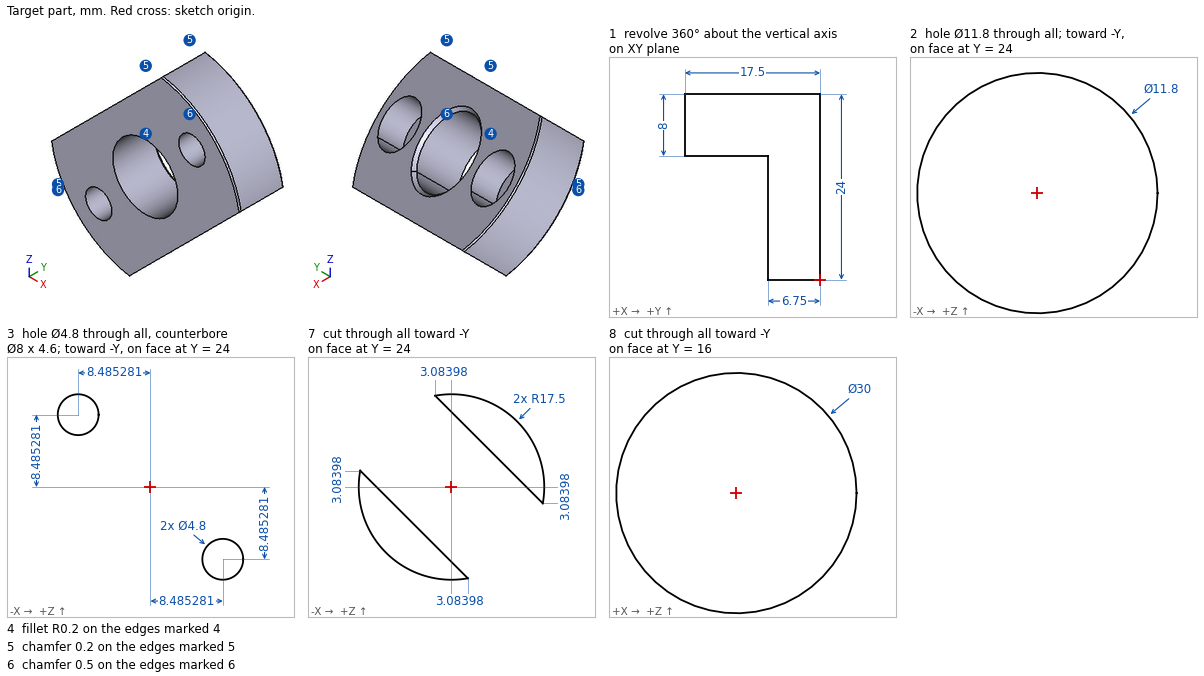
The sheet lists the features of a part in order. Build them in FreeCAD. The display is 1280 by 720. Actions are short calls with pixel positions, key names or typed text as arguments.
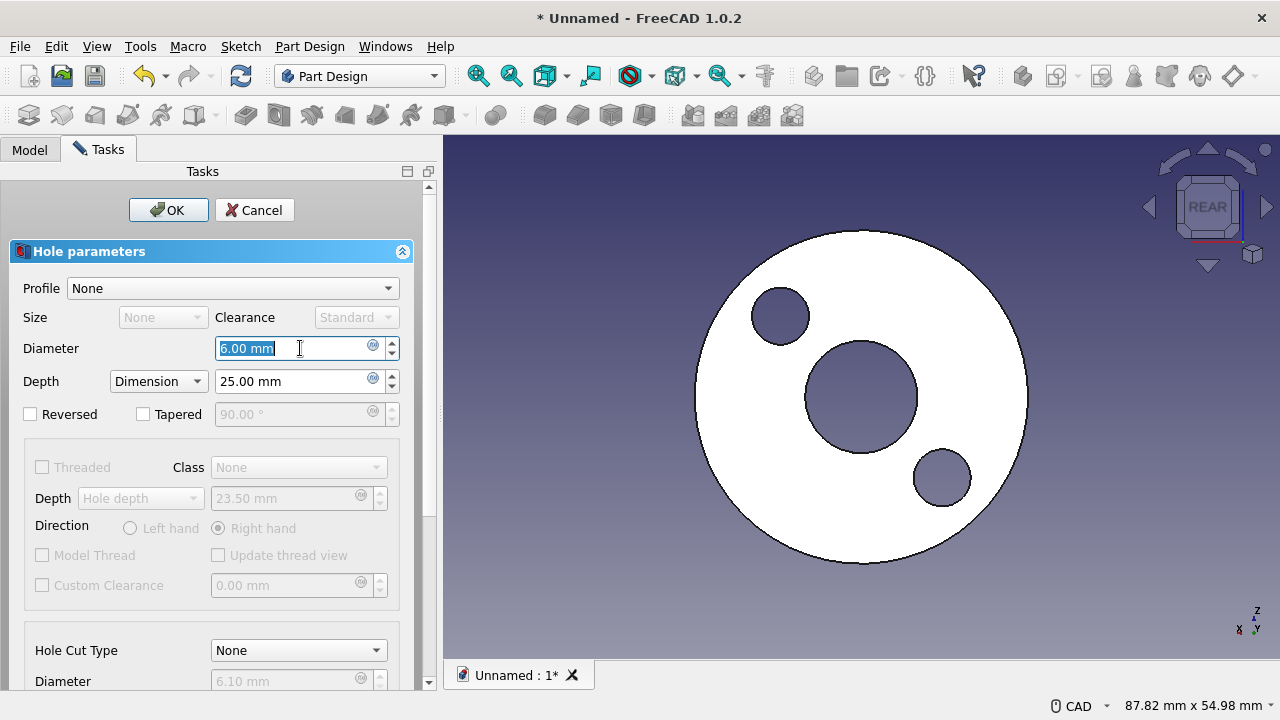
text(4.8)
key(Tab)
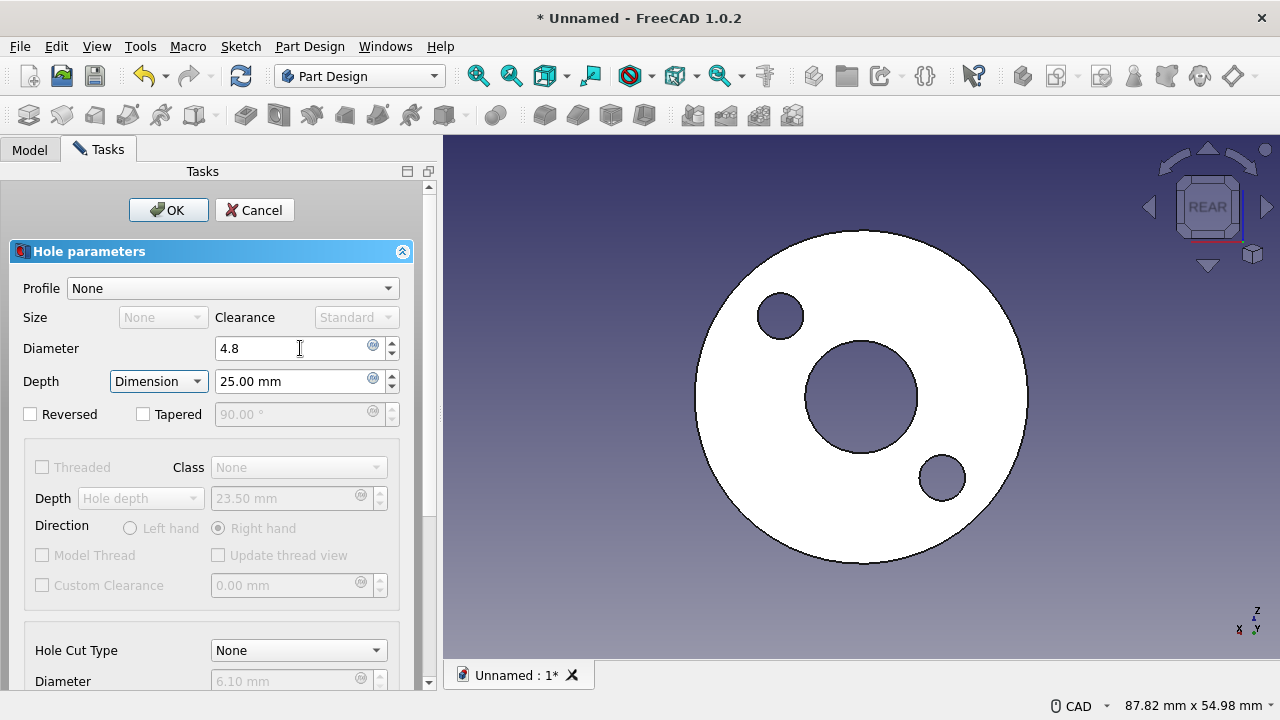
click(160, 382)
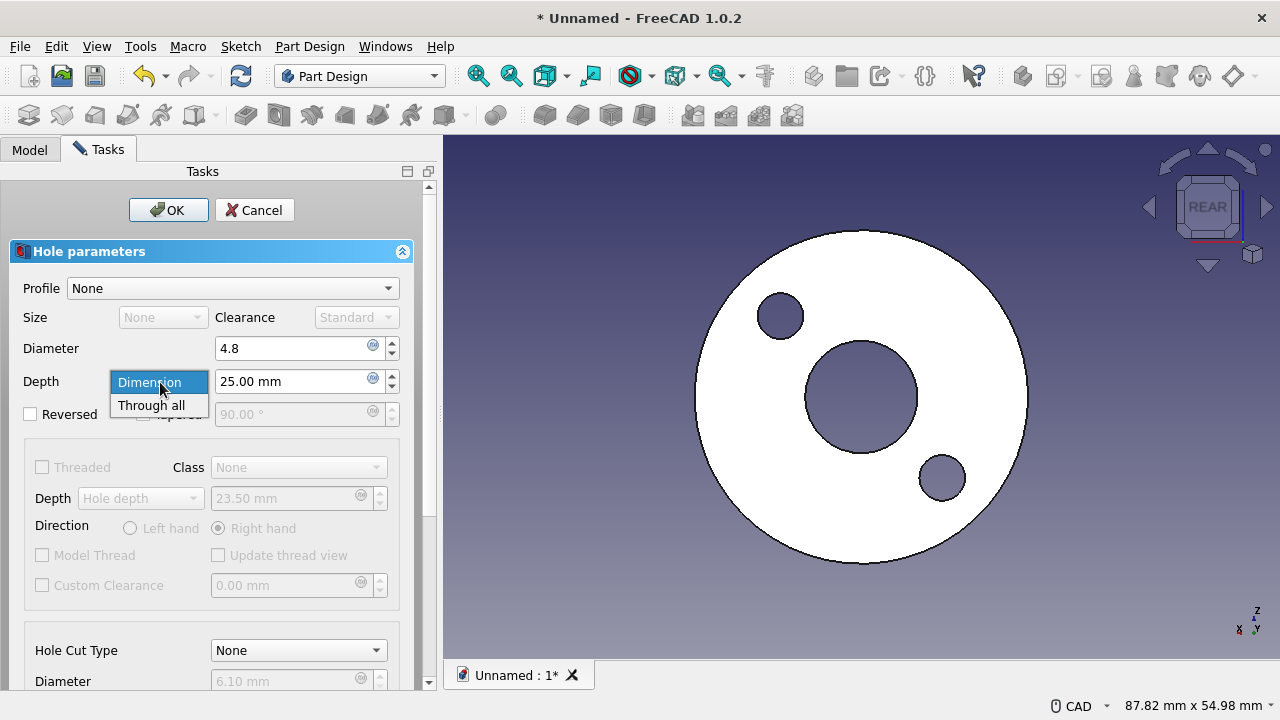
click(158, 406)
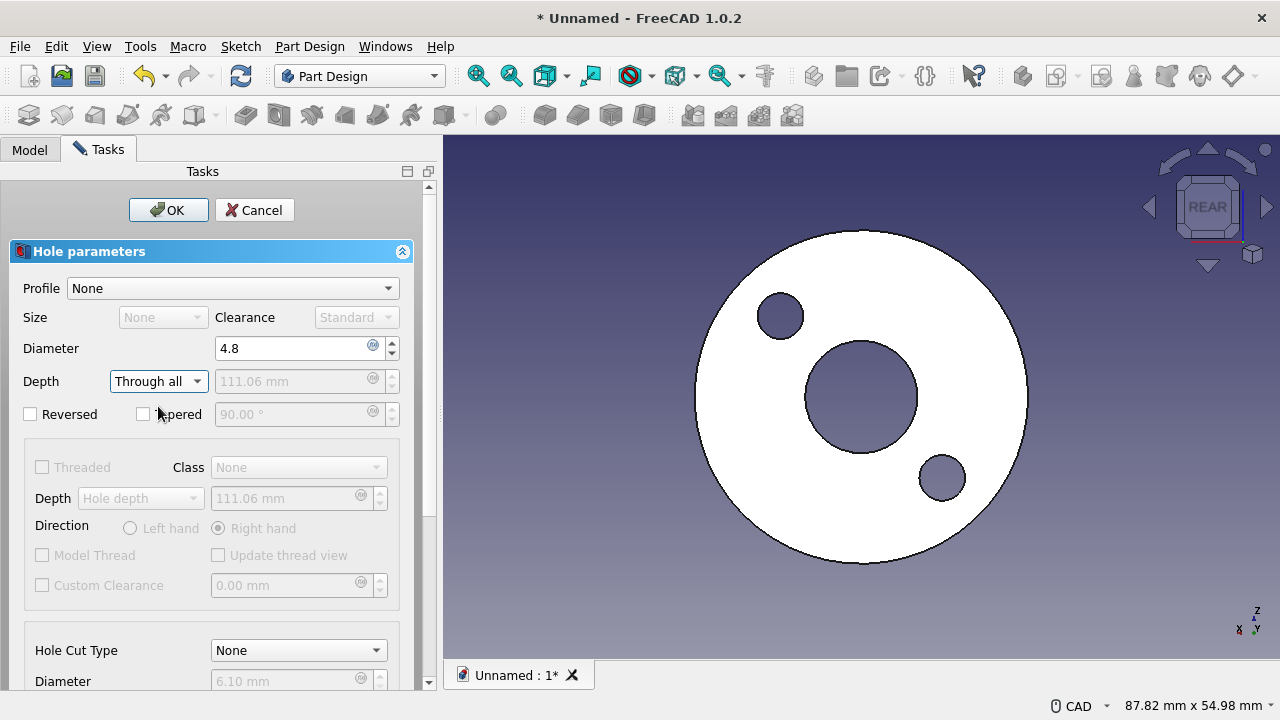
click(300, 650)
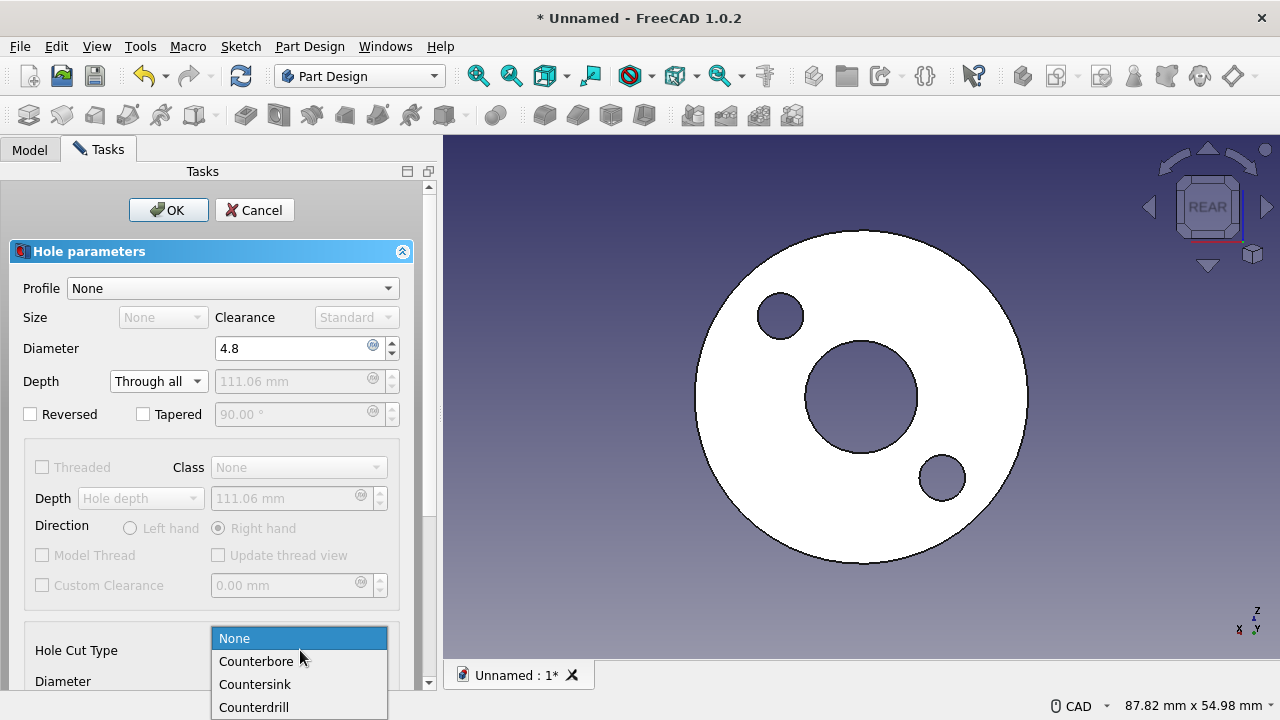
click(298, 662)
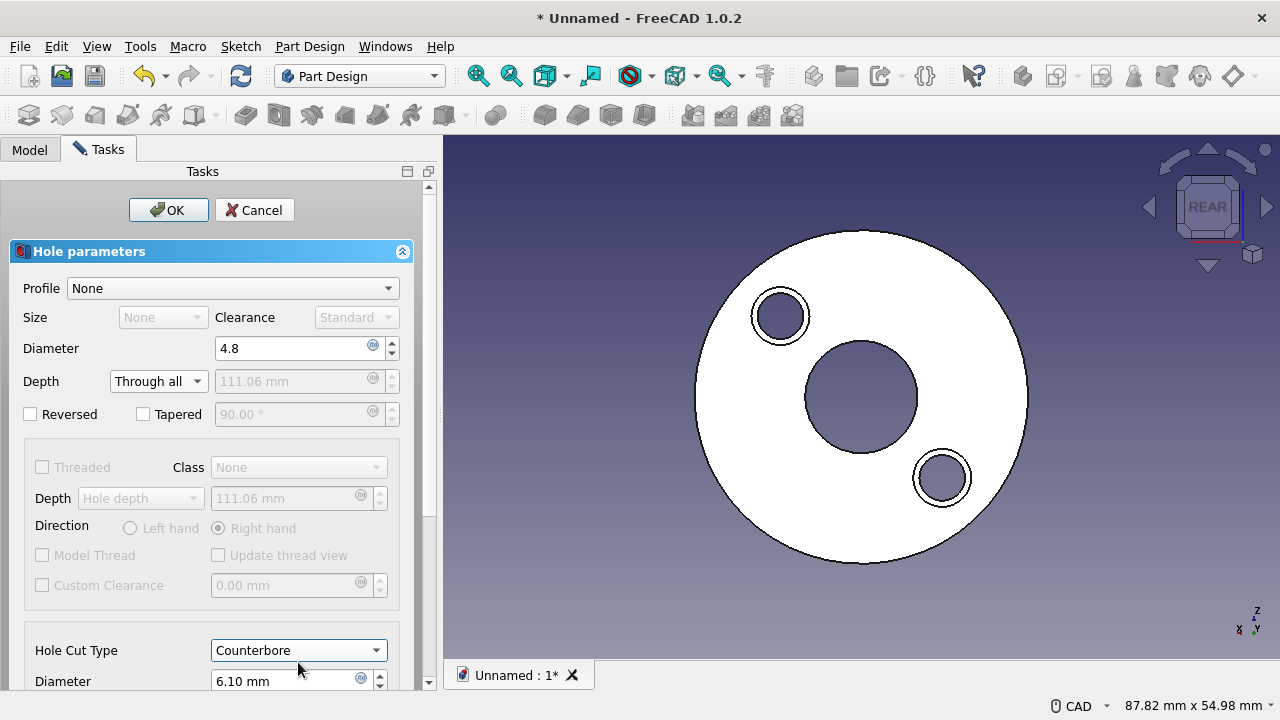
scroll(429, 436, down, 2)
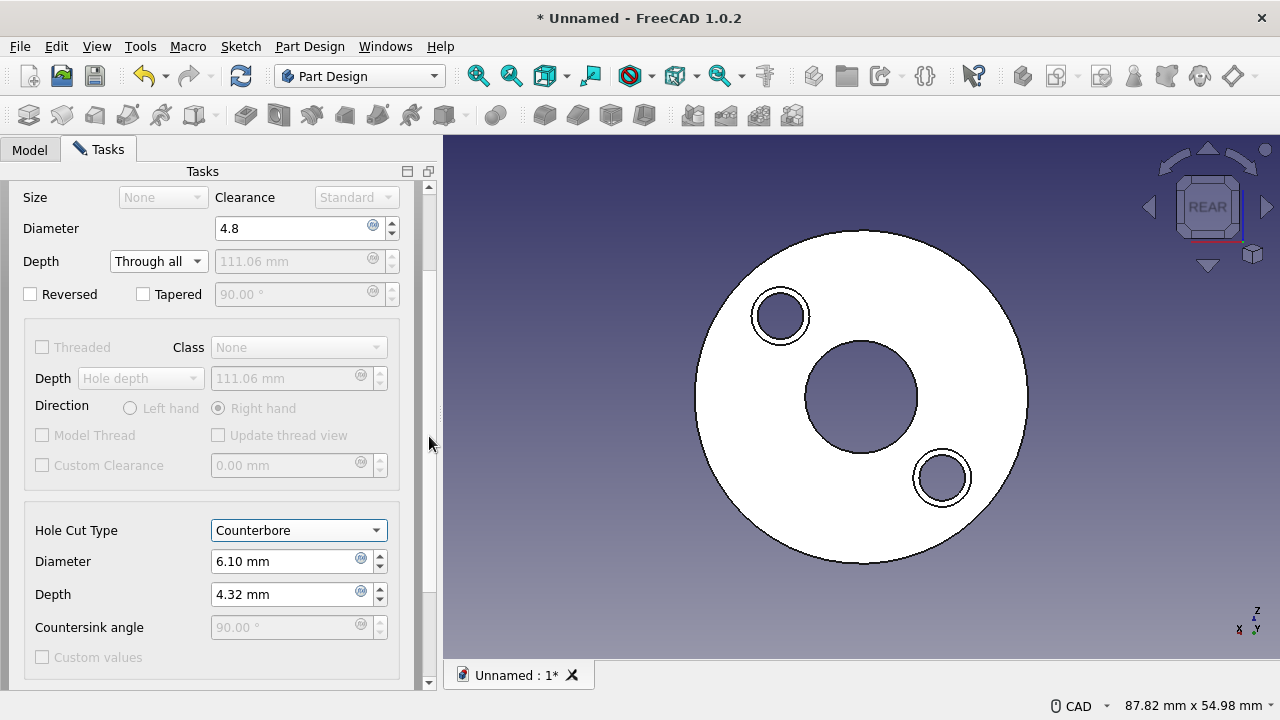
triple_click(292, 562)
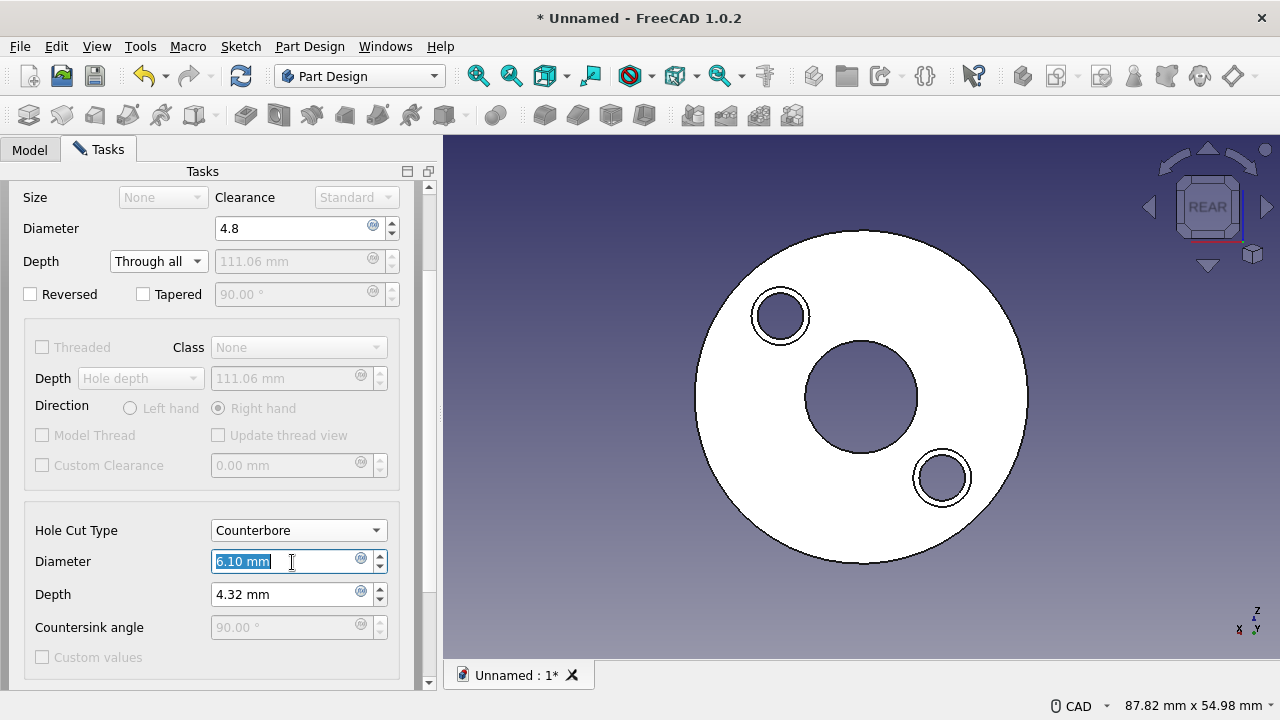
text(8)
key(Tab)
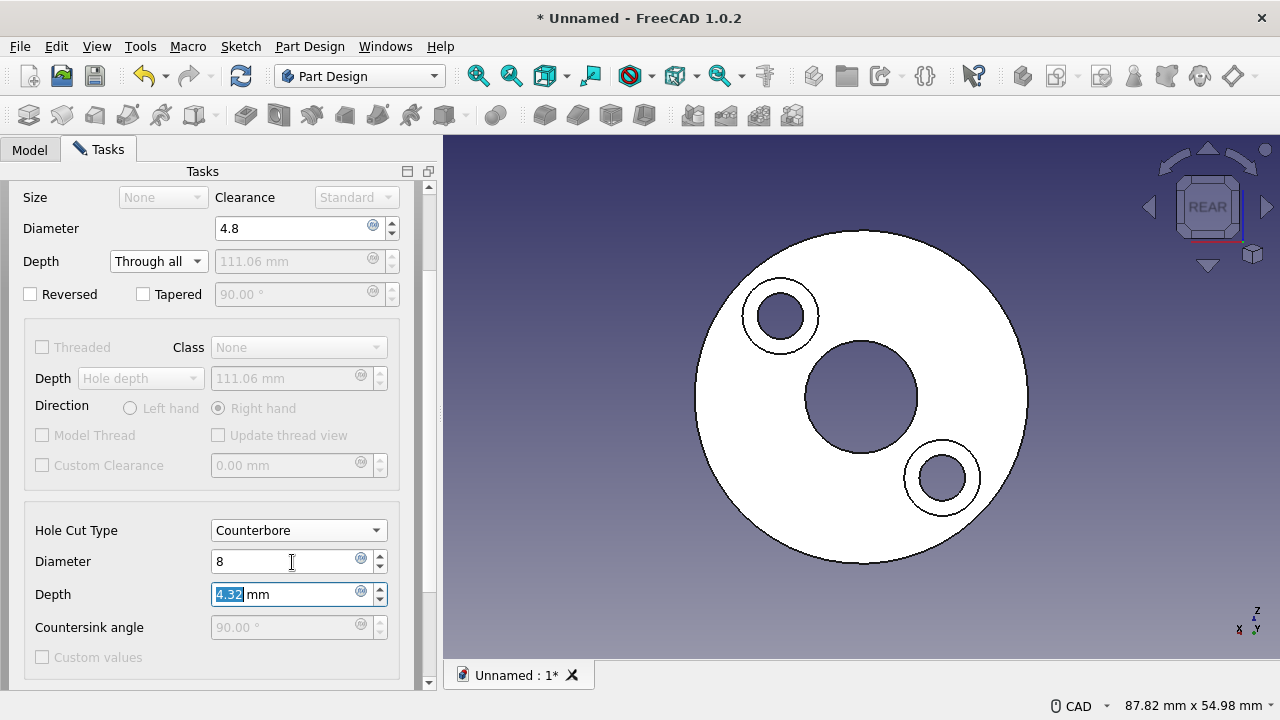
text(4.6)
key(Tab)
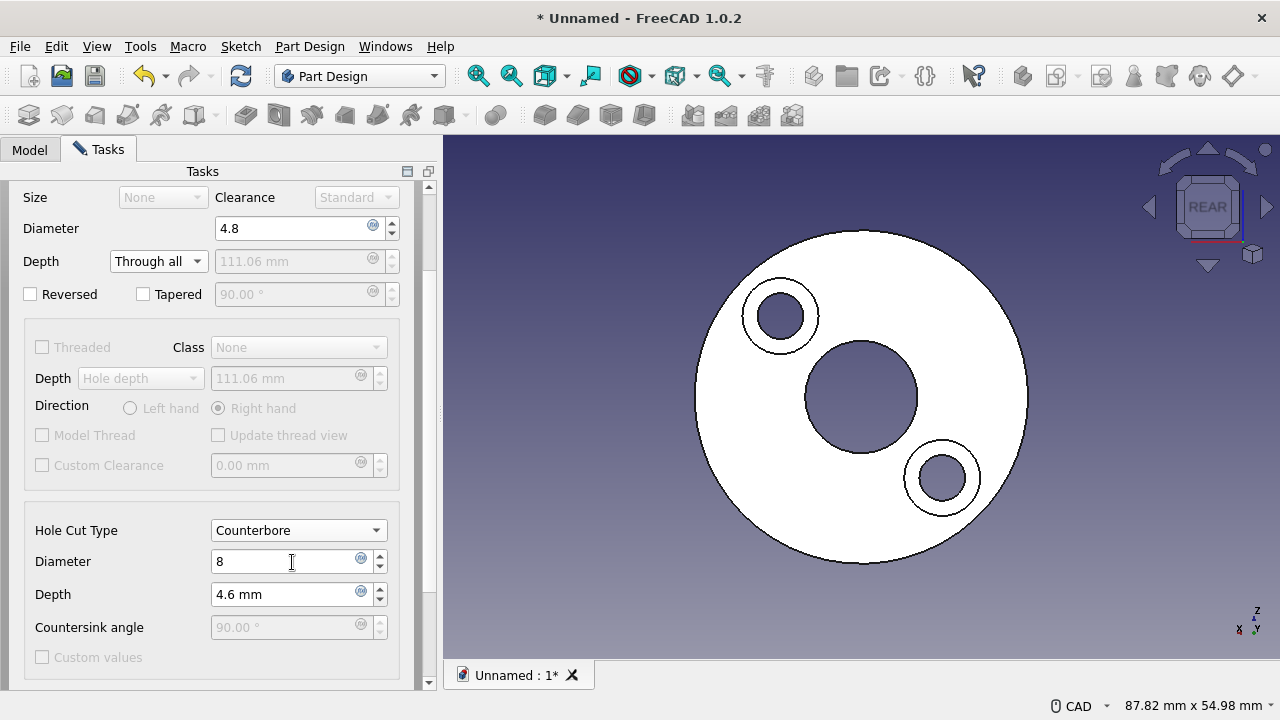
scroll(429, 436, up, 3)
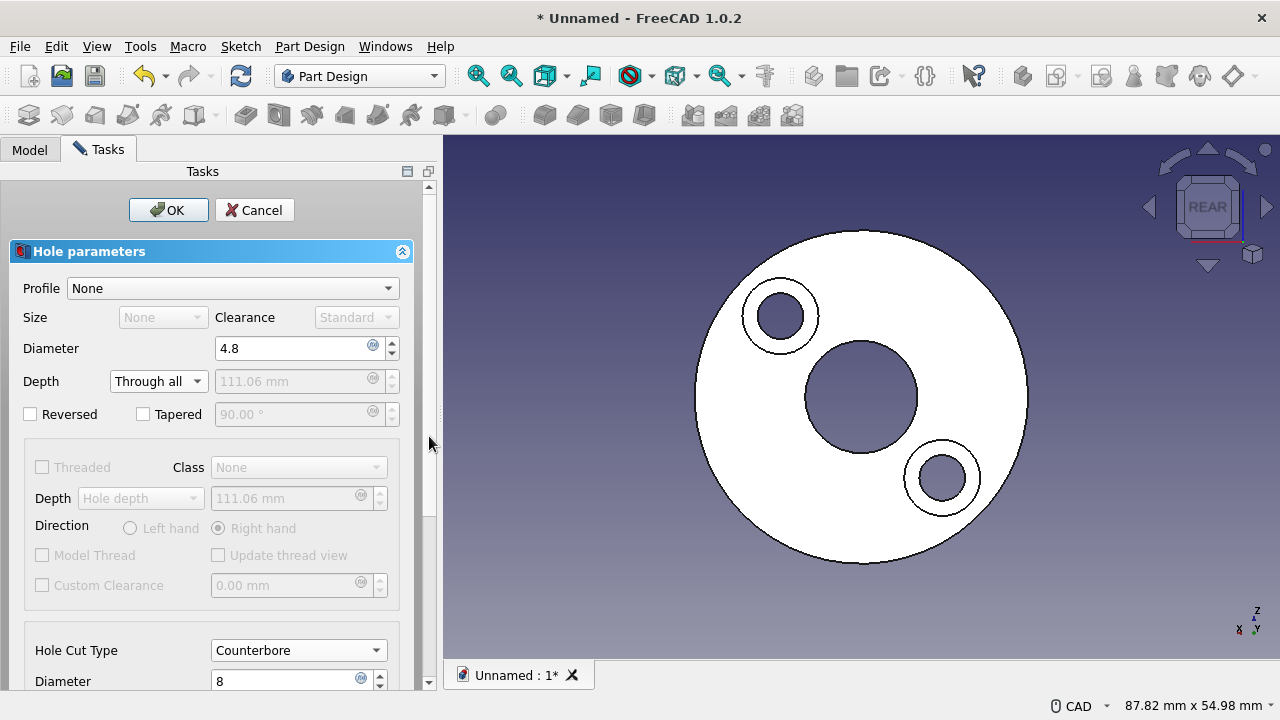
click(169, 210)